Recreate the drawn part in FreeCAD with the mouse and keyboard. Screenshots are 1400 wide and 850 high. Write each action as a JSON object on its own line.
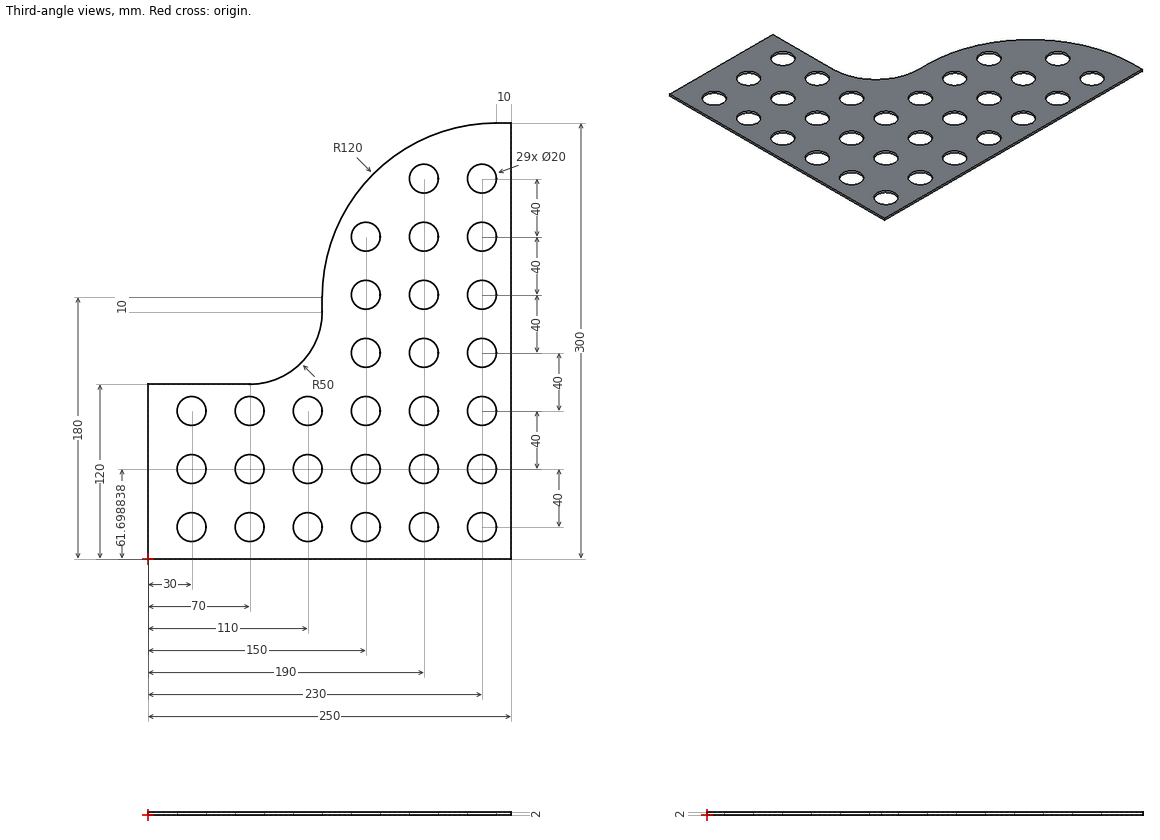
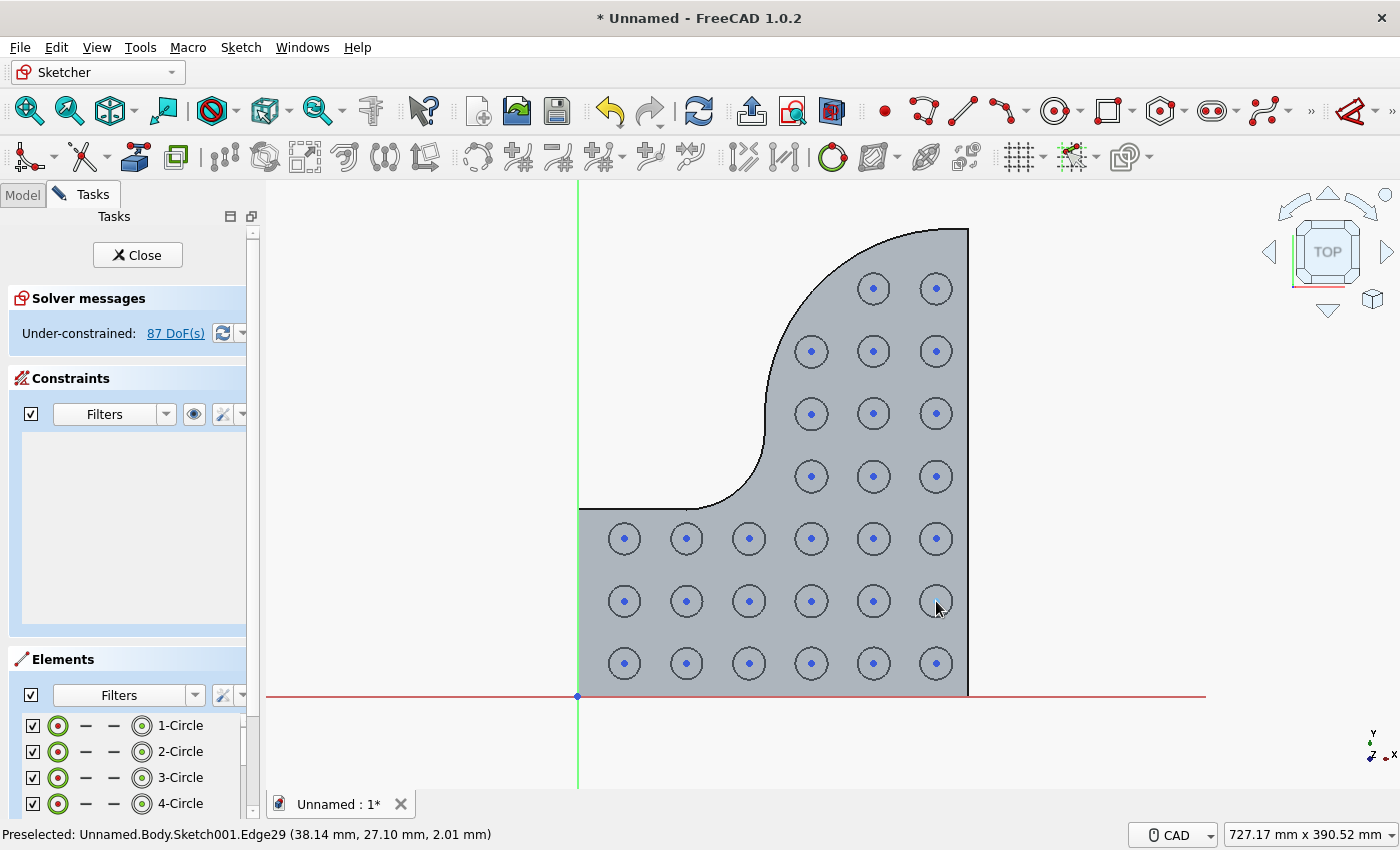
{"action": "left_click", "coordinate": [947, 278]}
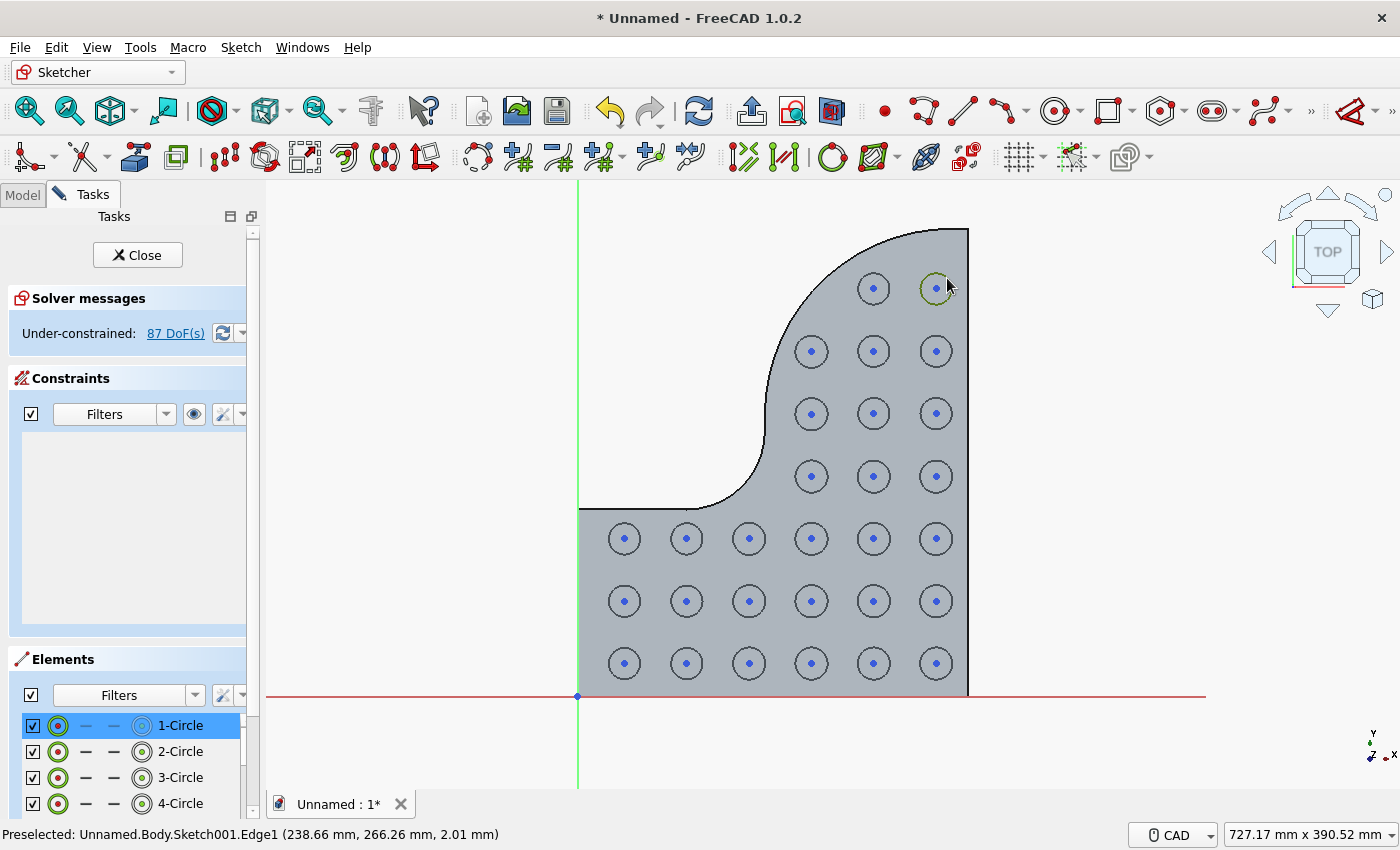
{"action": "left_click", "coordinate": [885, 278]}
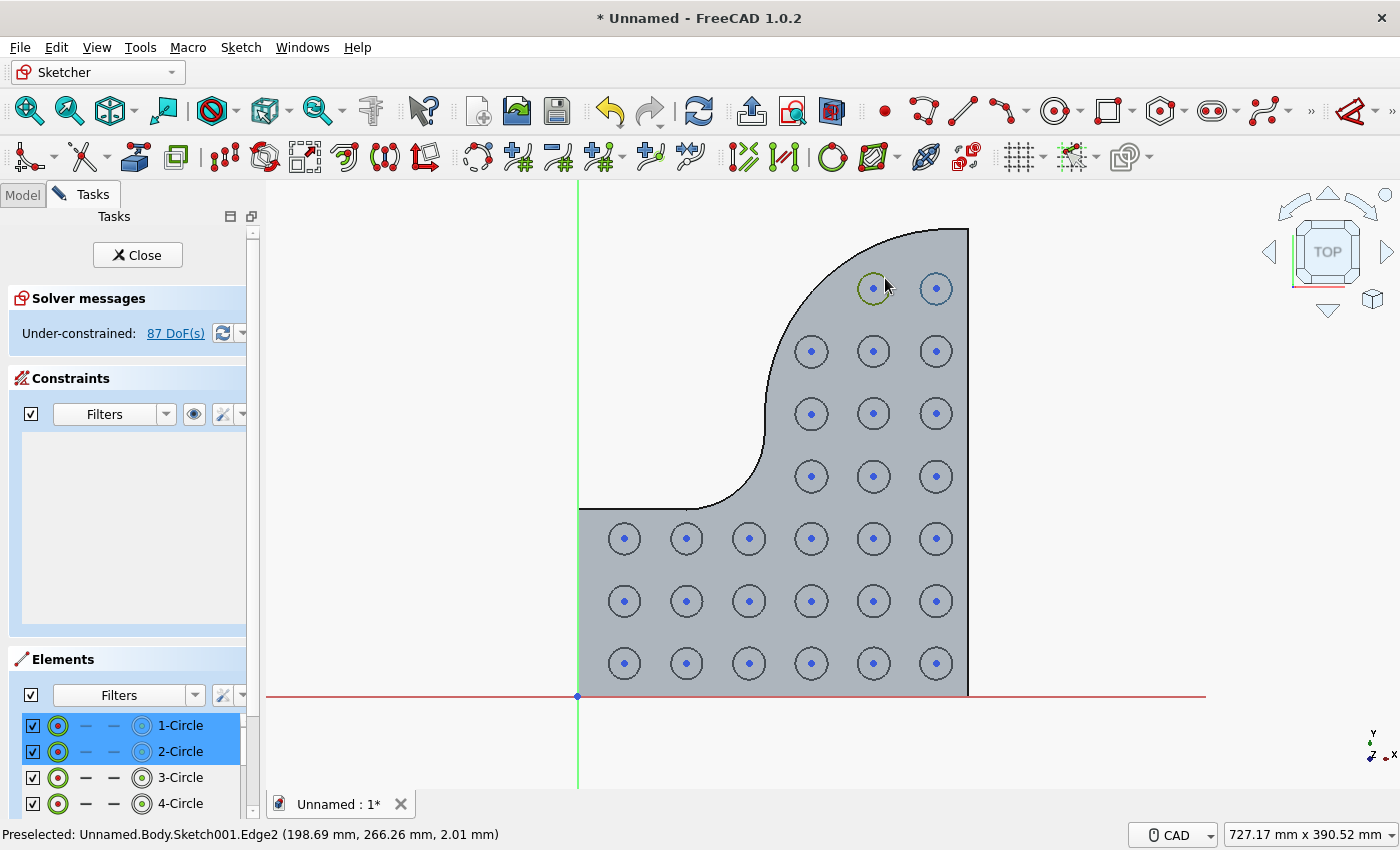
{"action": "left_click", "coordinate": [947, 340]}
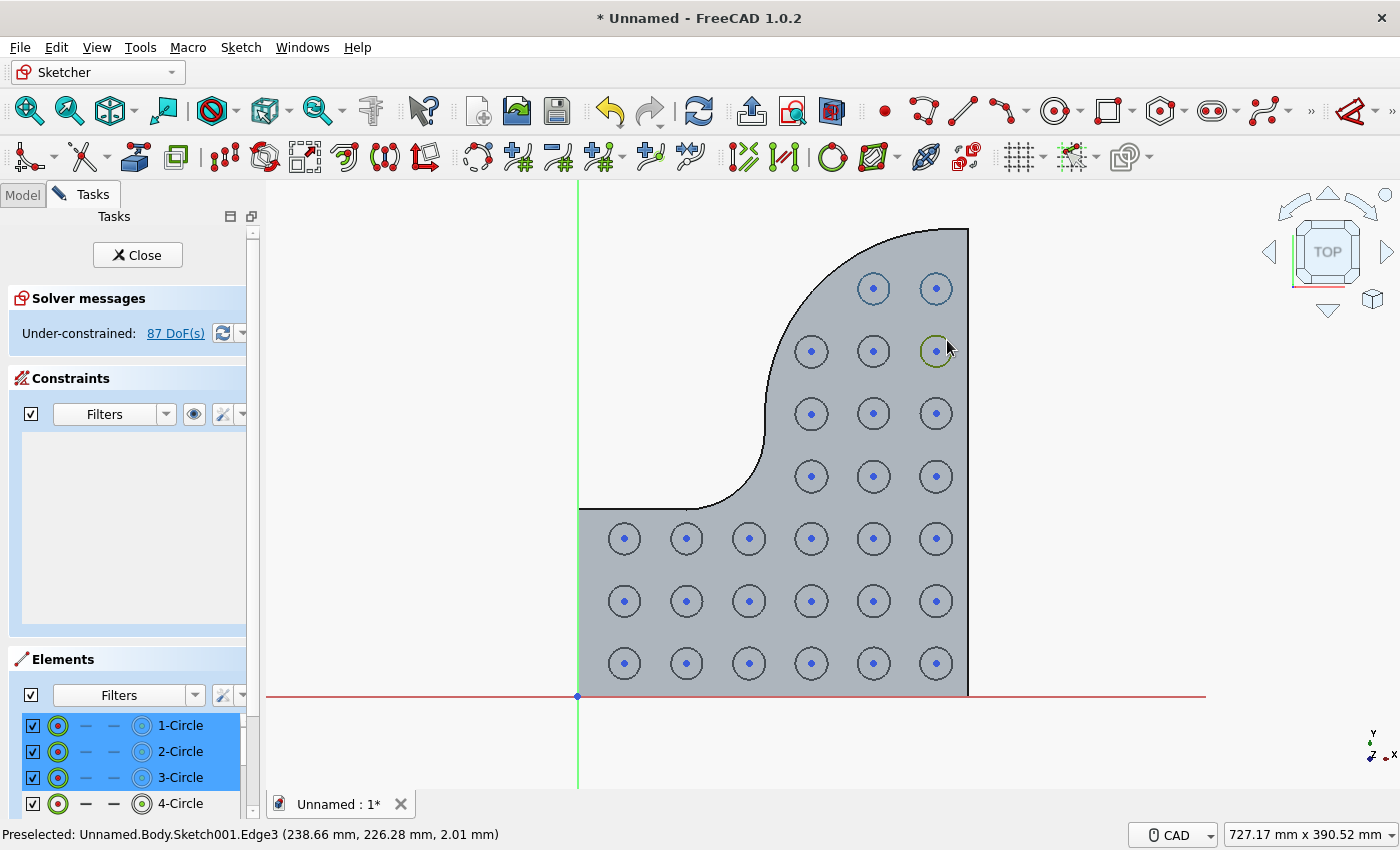
{"action": "left_click", "coordinate": [885, 340]}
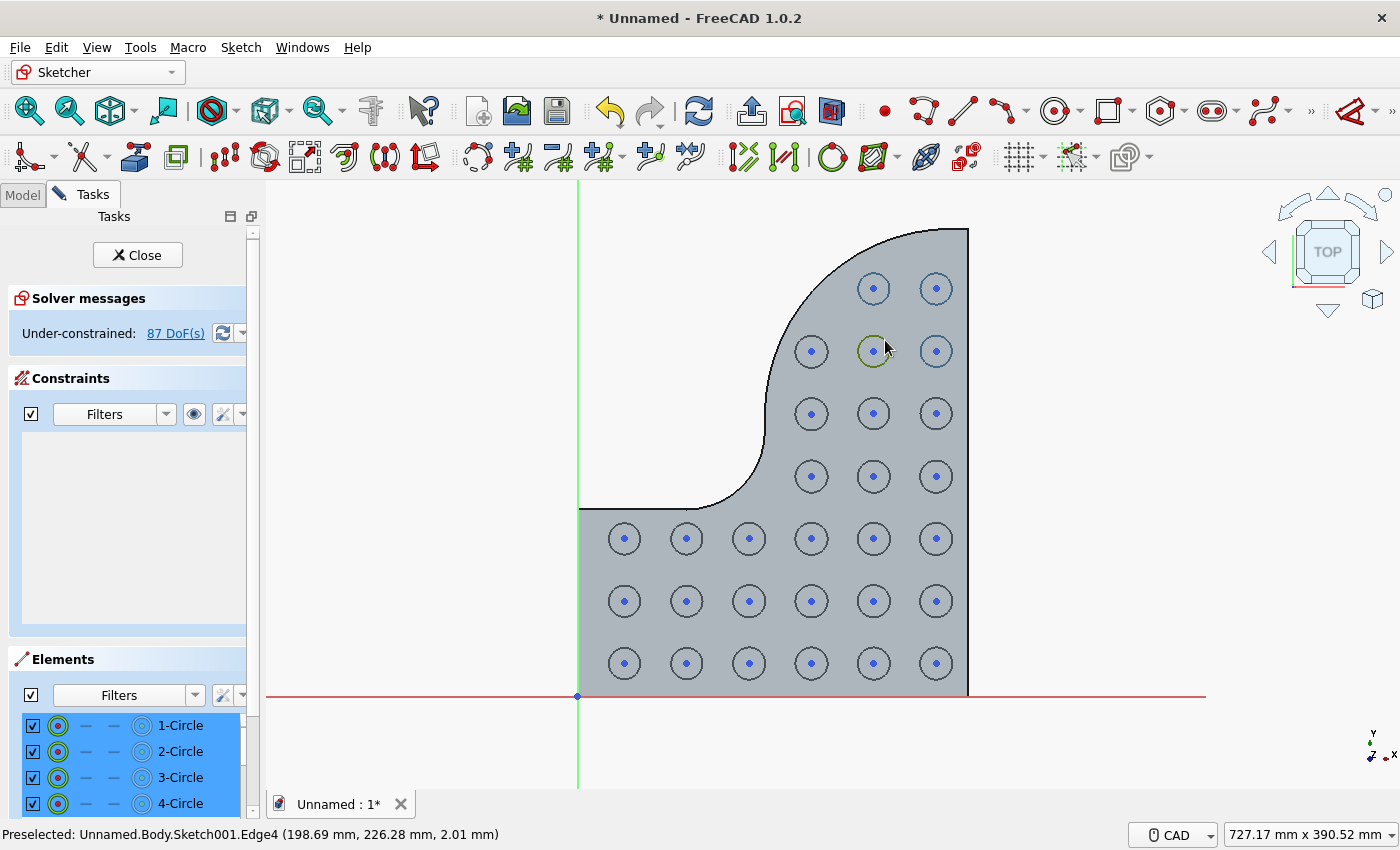
{"action": "left_click", "coordinate": [947, 403]}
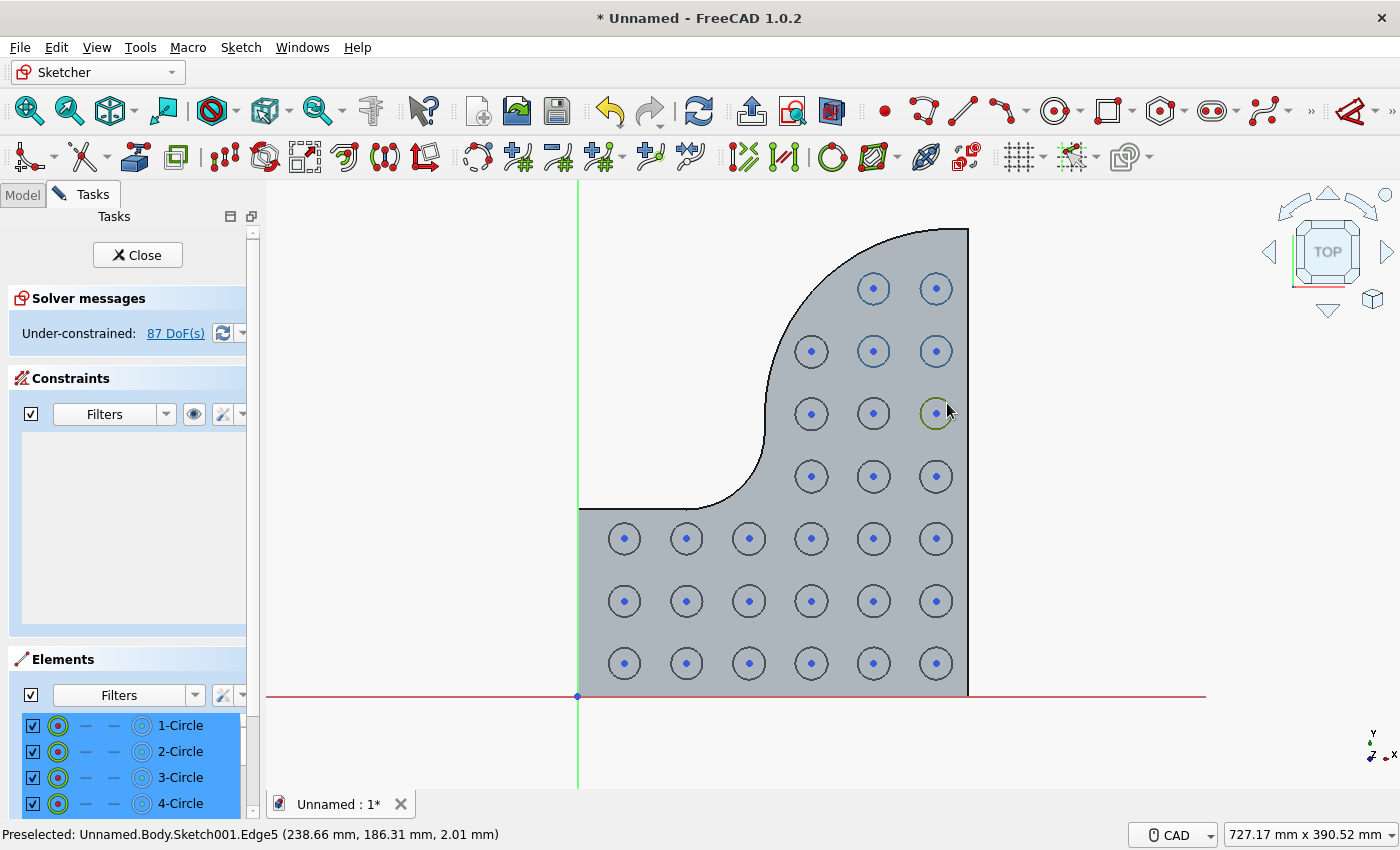
{"action": "left_click", "coordinate": [885, 403]}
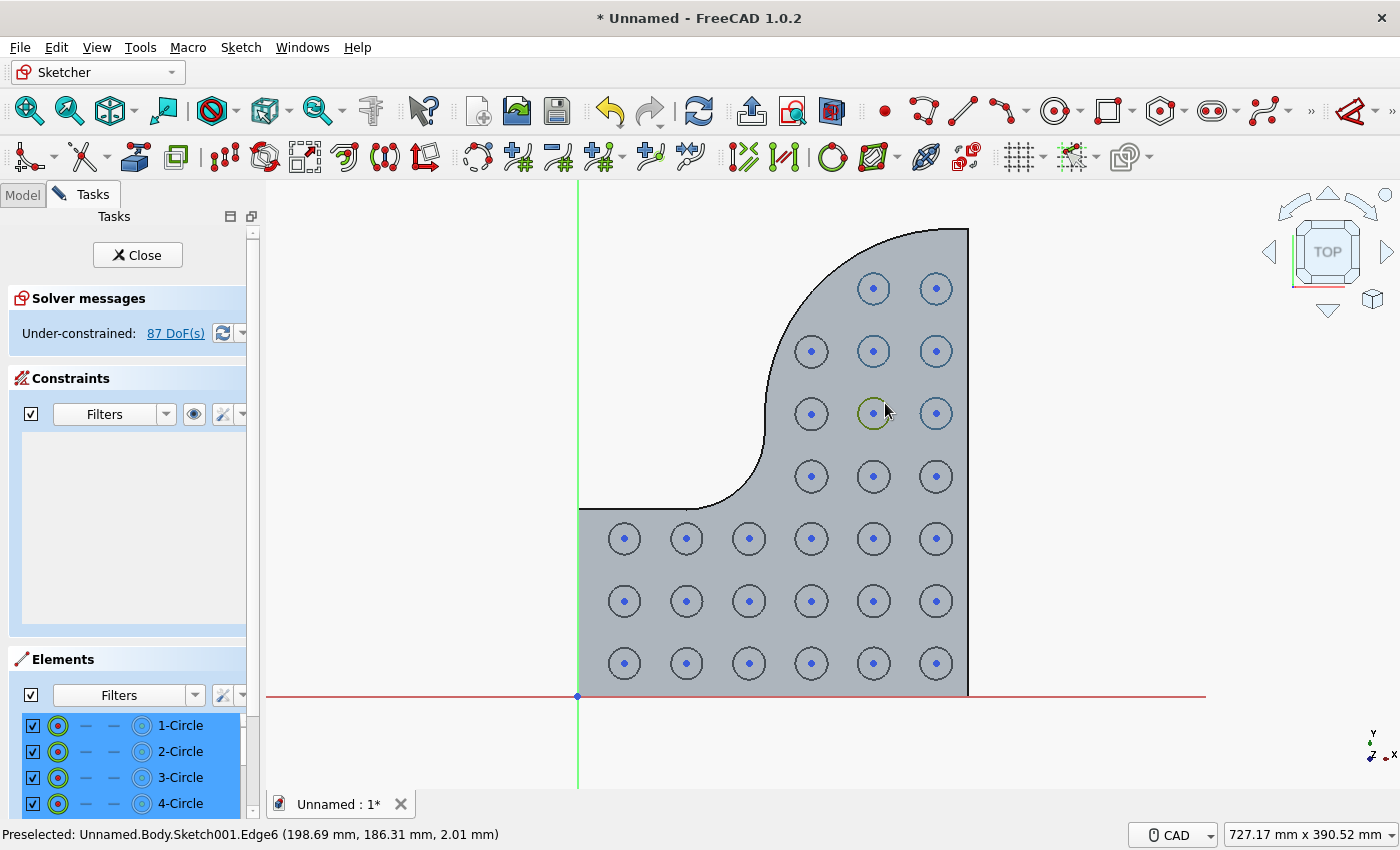
{"action": "left_click", "coordinate": [948, 465]}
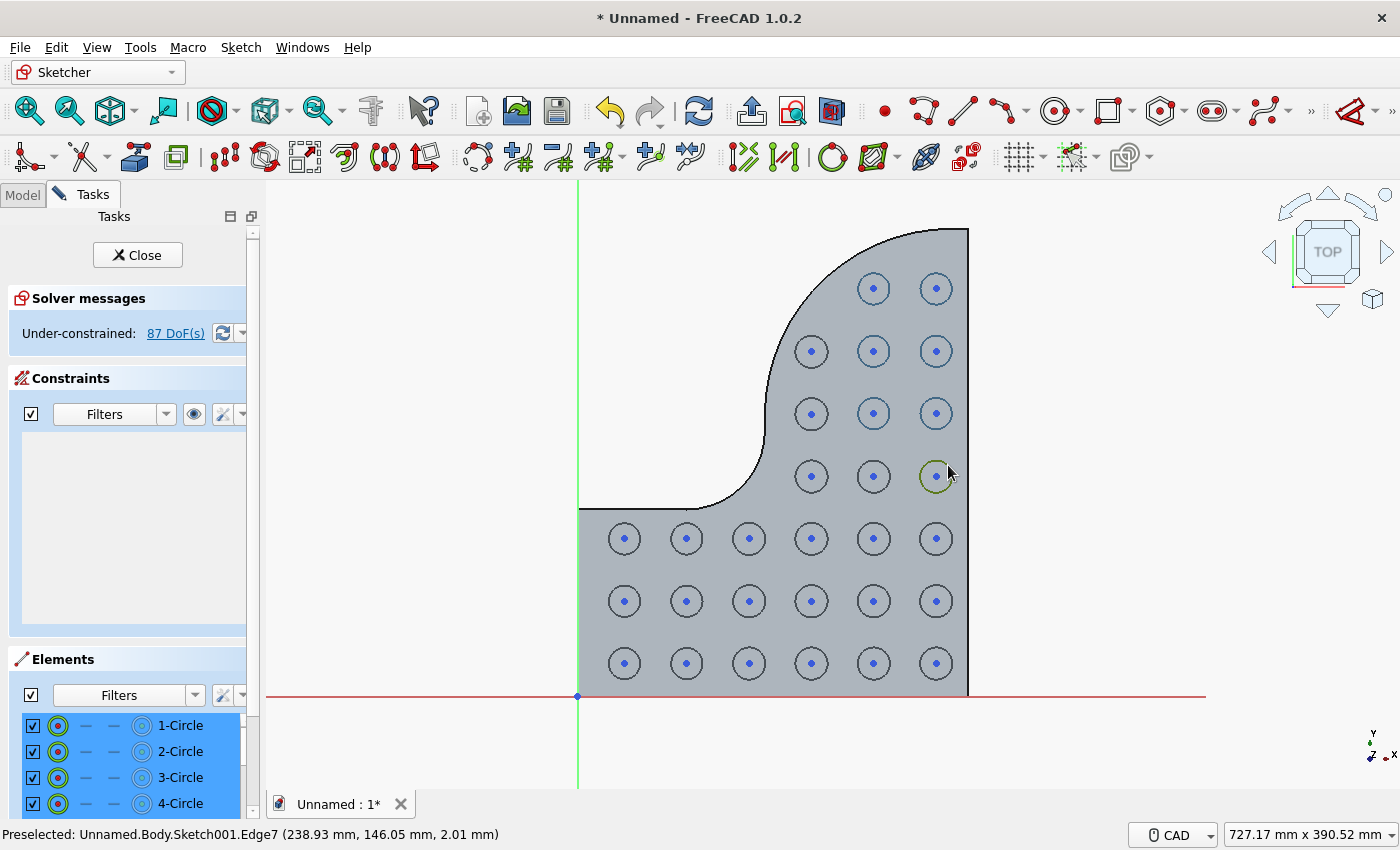
{"action": "left_click", "coordinate": [885, 465]}